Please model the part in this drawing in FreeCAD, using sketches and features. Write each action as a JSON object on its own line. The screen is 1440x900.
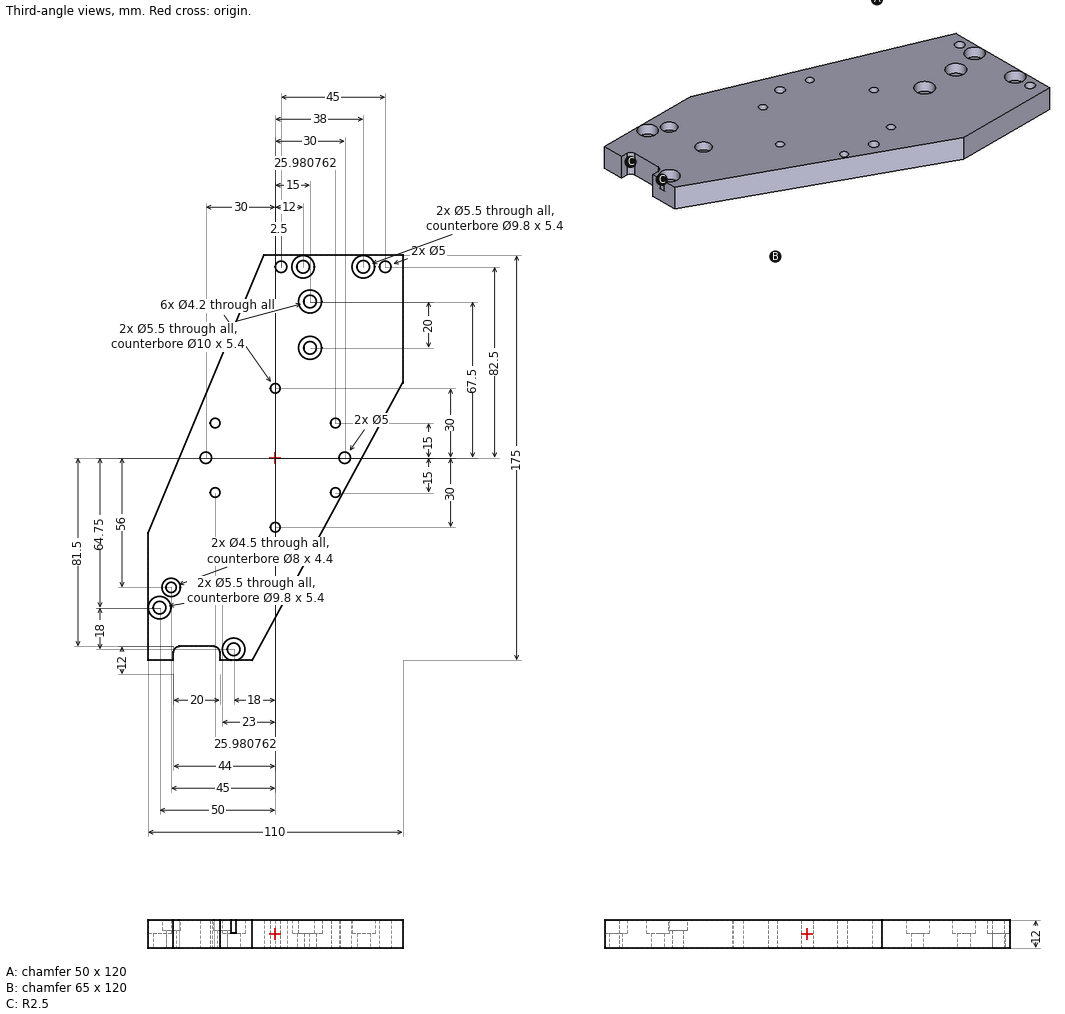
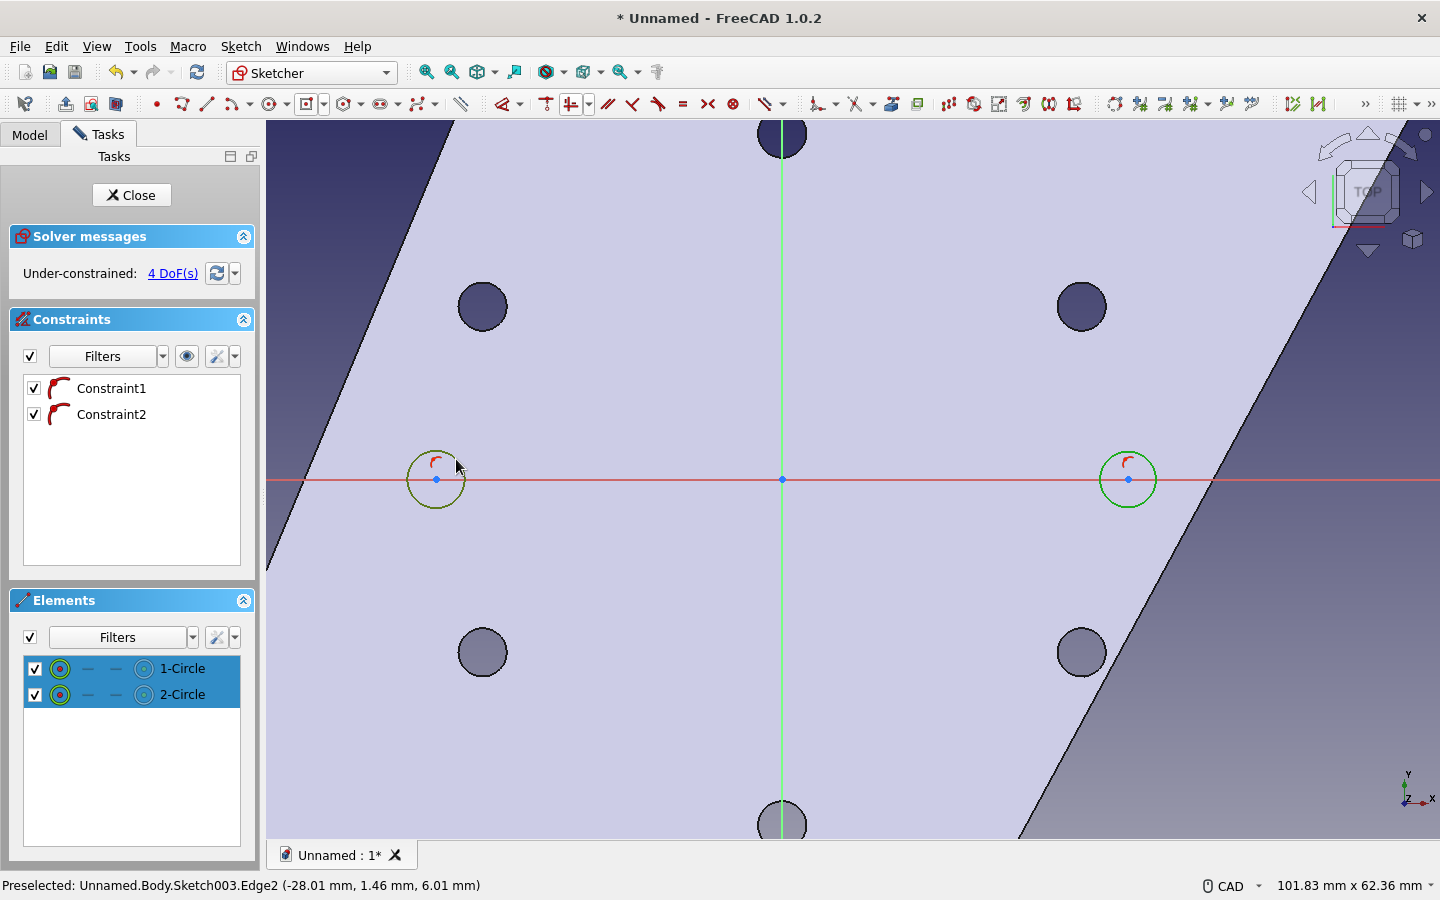
{"action": "left_click", "coordinate": [683, 104]}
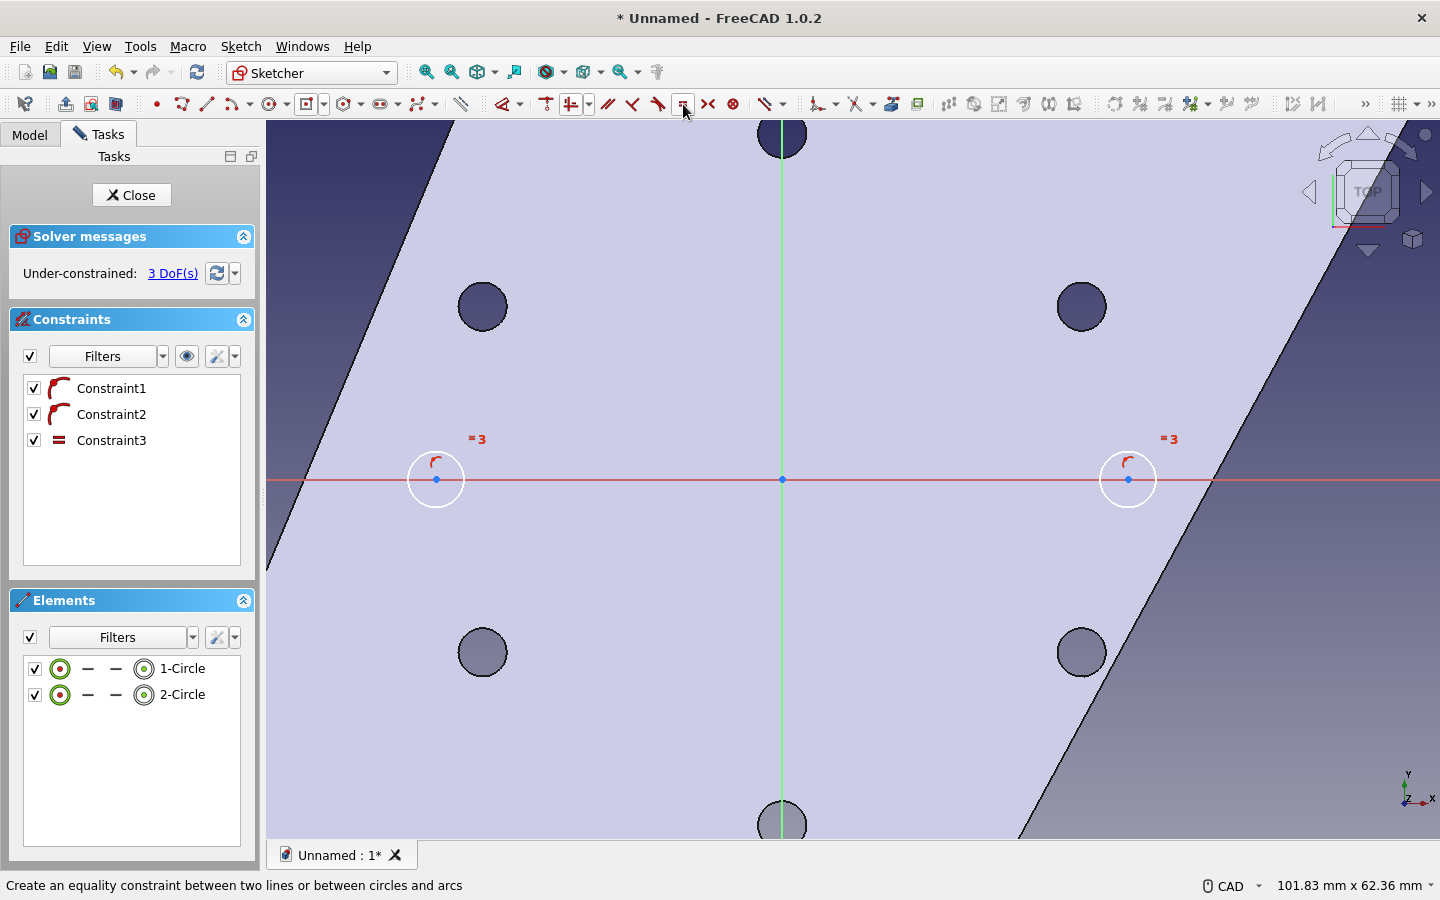
{"action": "left_click", "coordinate": [1148, 460]}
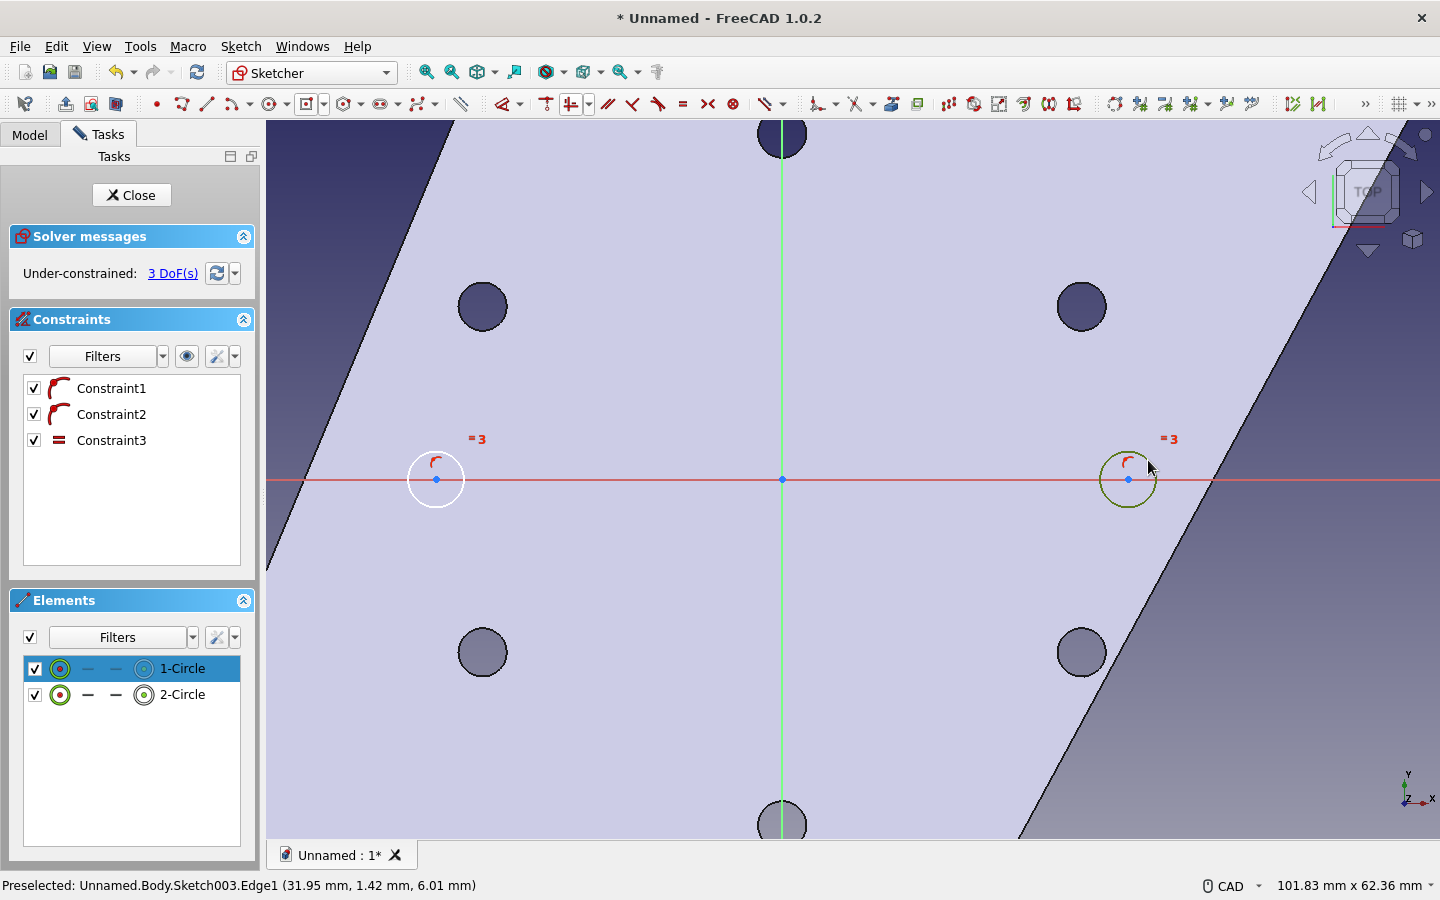
{"action": "key", "text": "k o"}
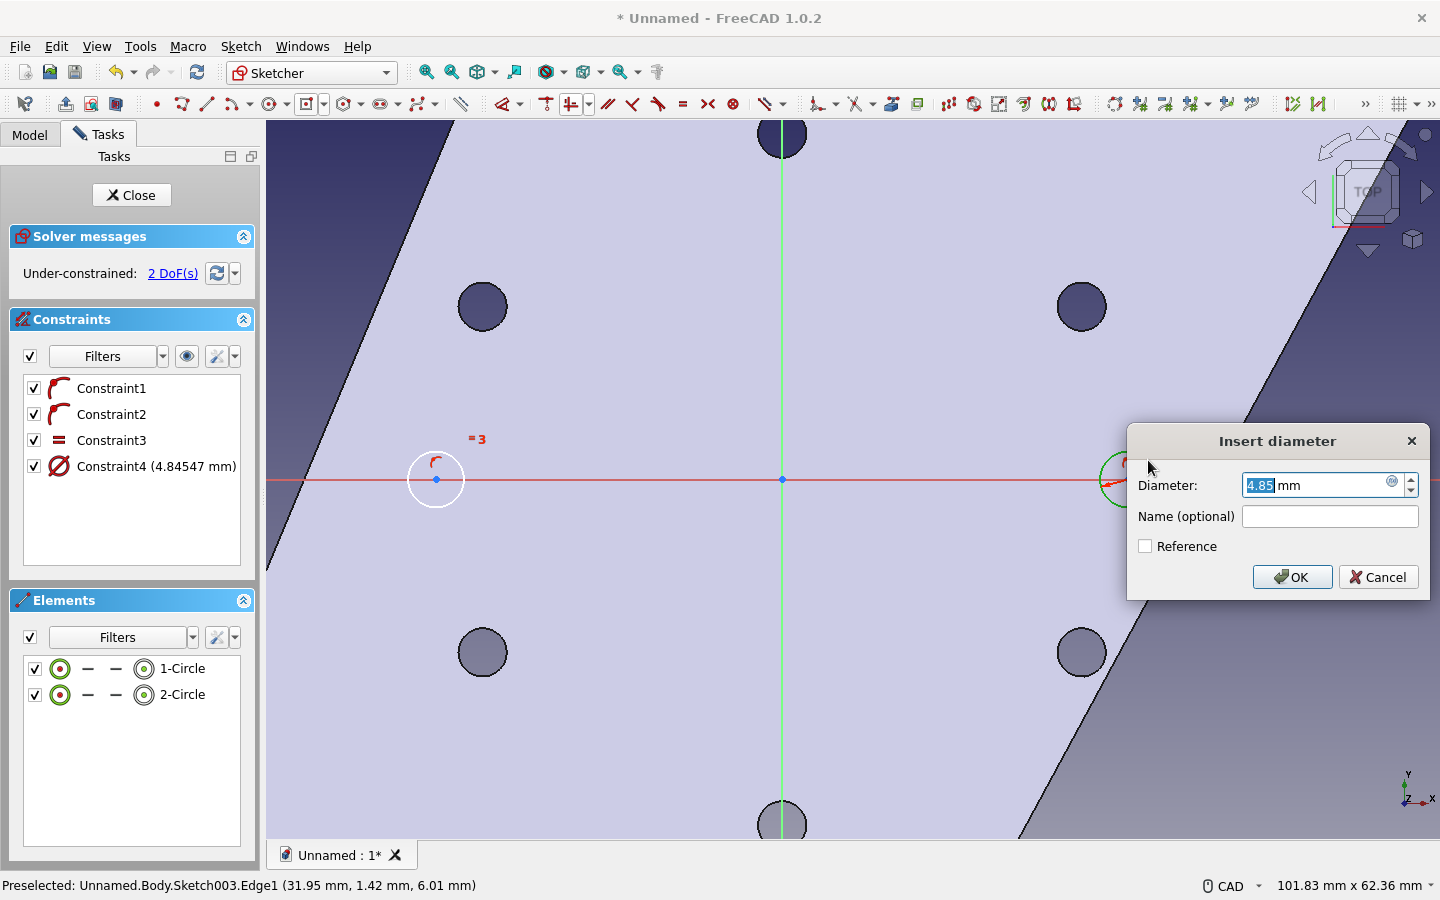
{"action": "type", "text": "5"}
{"action": "key", "text": "Return"}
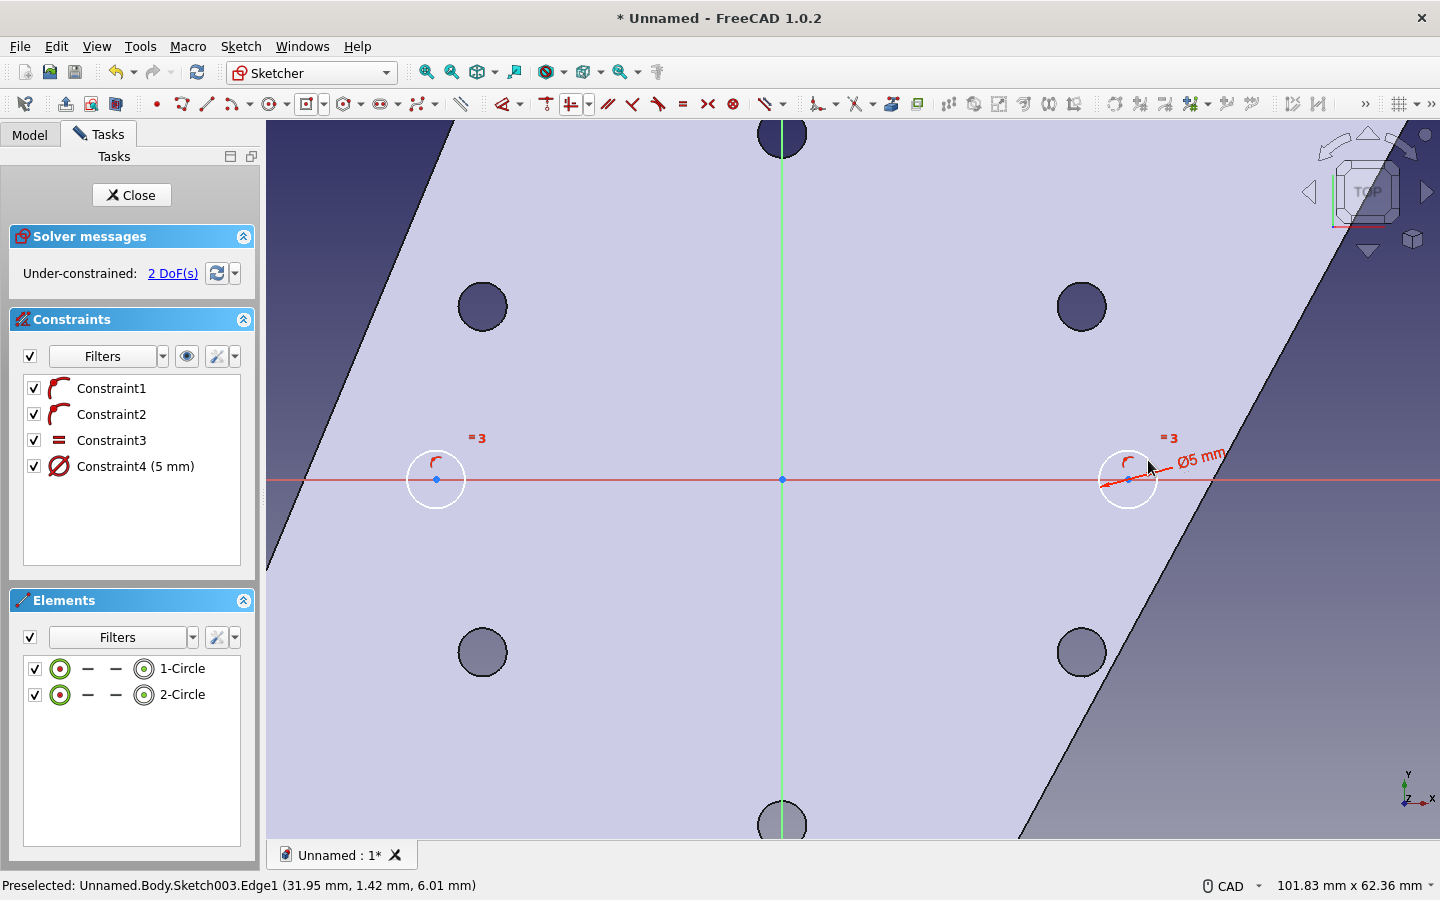
{"action": "left_click", "coordinate": [1128, 479]}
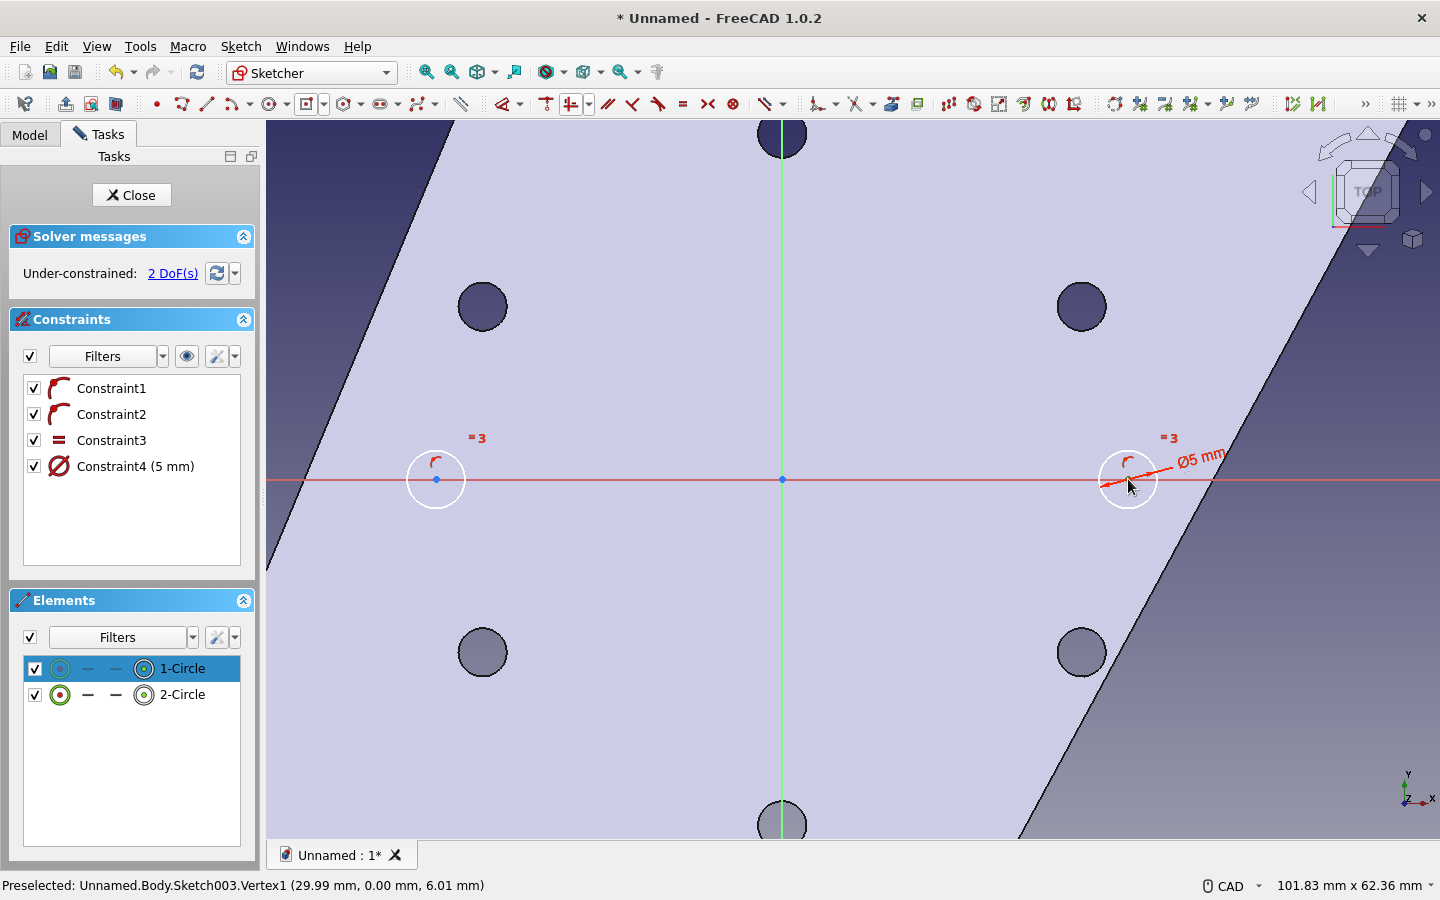
{"action": "left_click", "coordinate": [520, 104]}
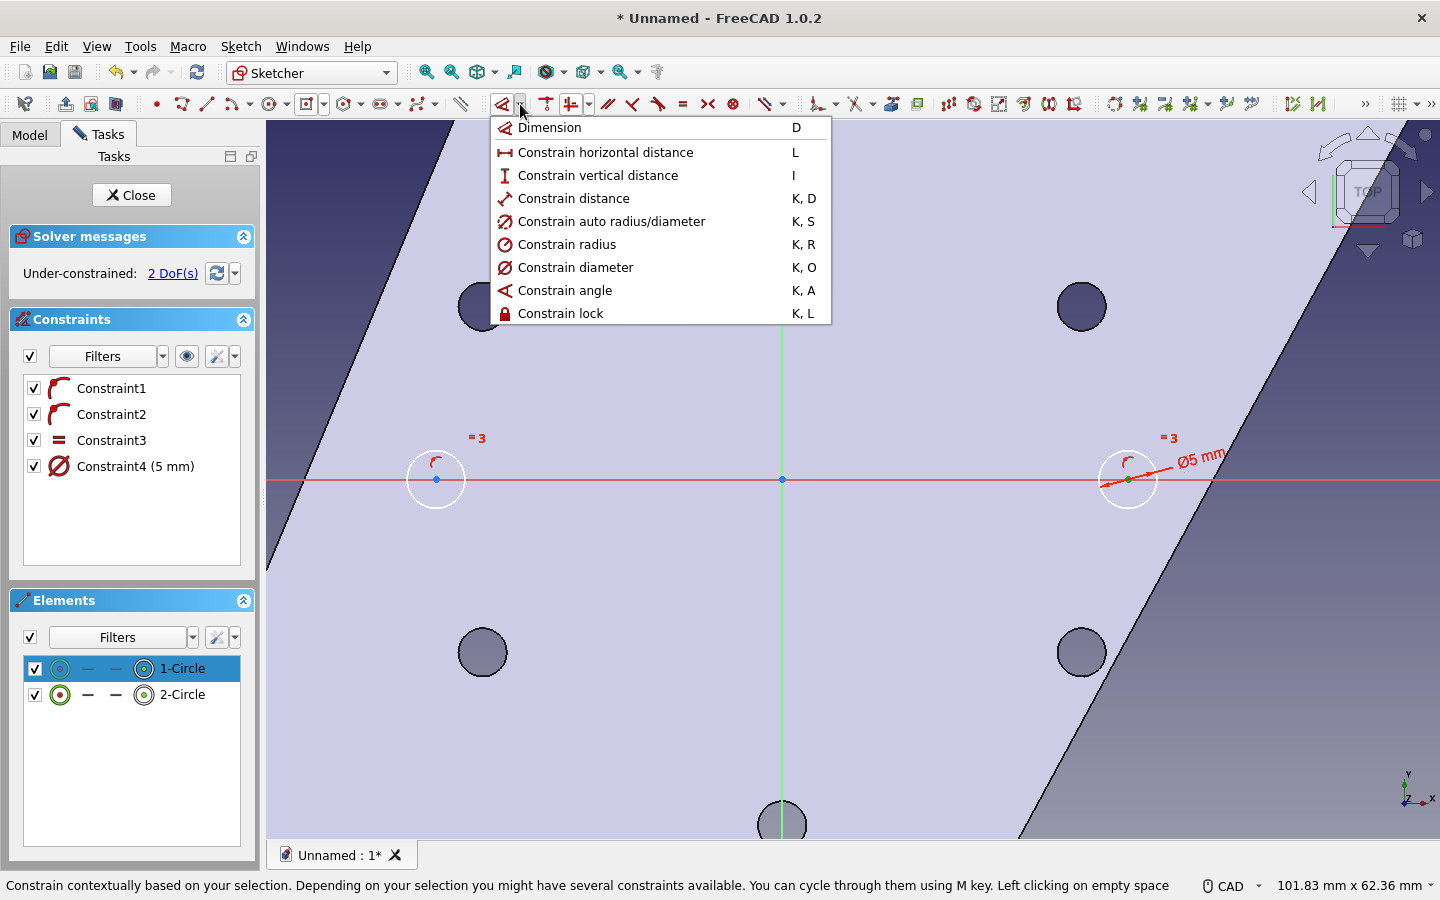
{"action": "left_click", "coordinate": [661, 152]}